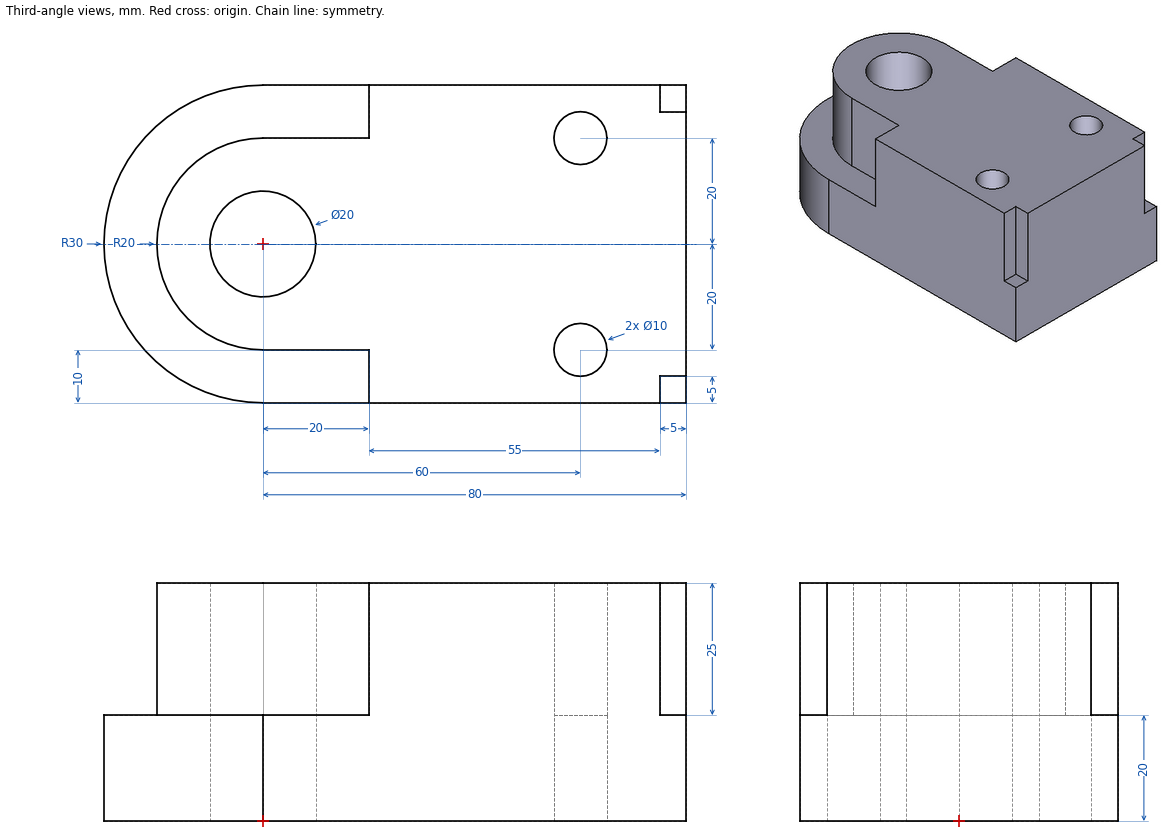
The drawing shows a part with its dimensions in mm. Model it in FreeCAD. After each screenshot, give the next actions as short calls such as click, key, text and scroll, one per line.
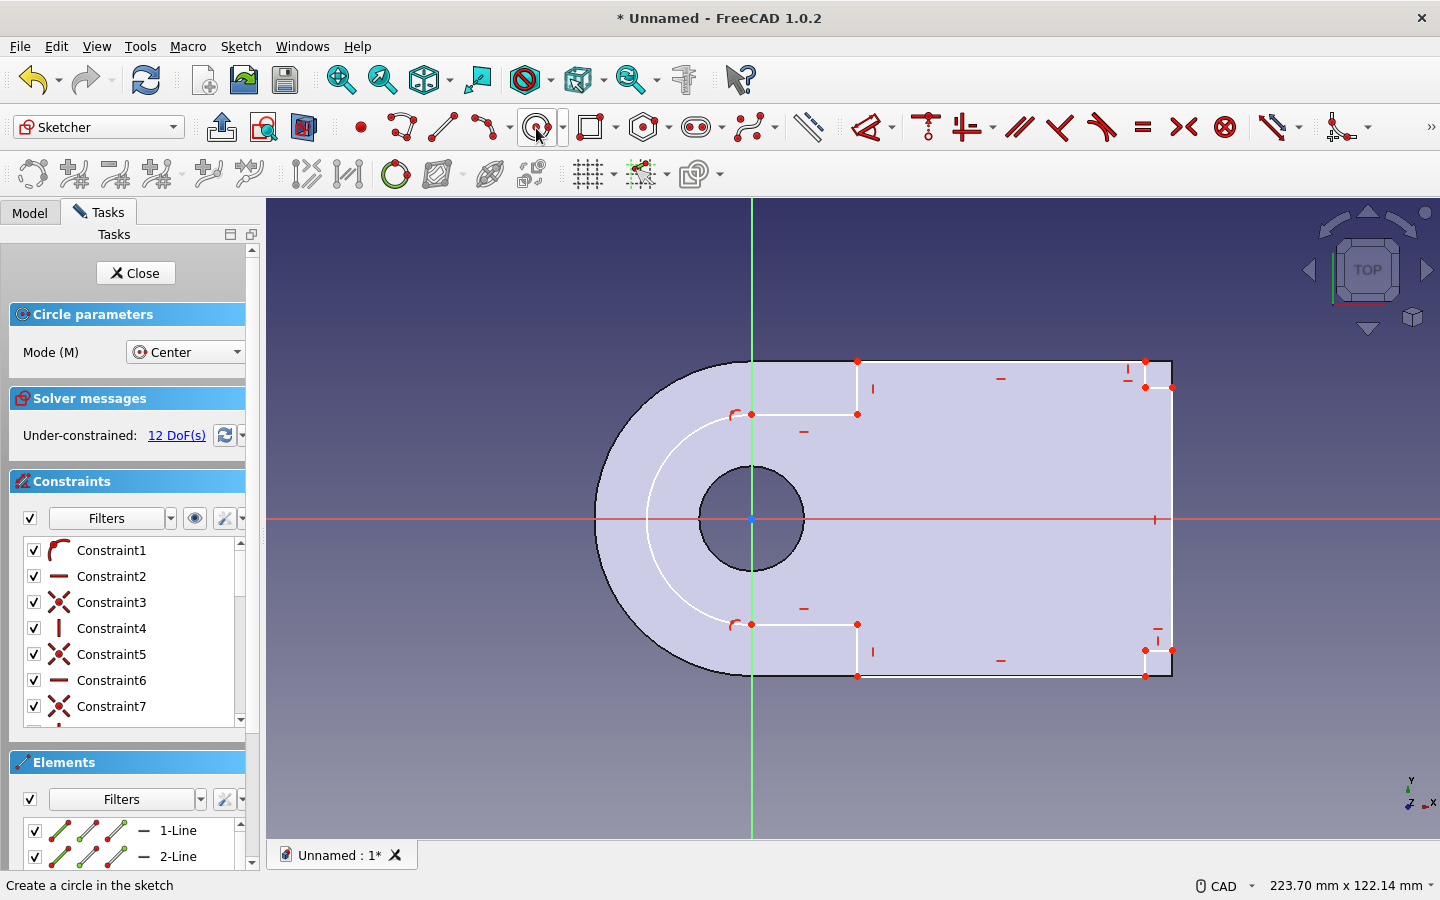
click(1067, 624)
move(1085, 605)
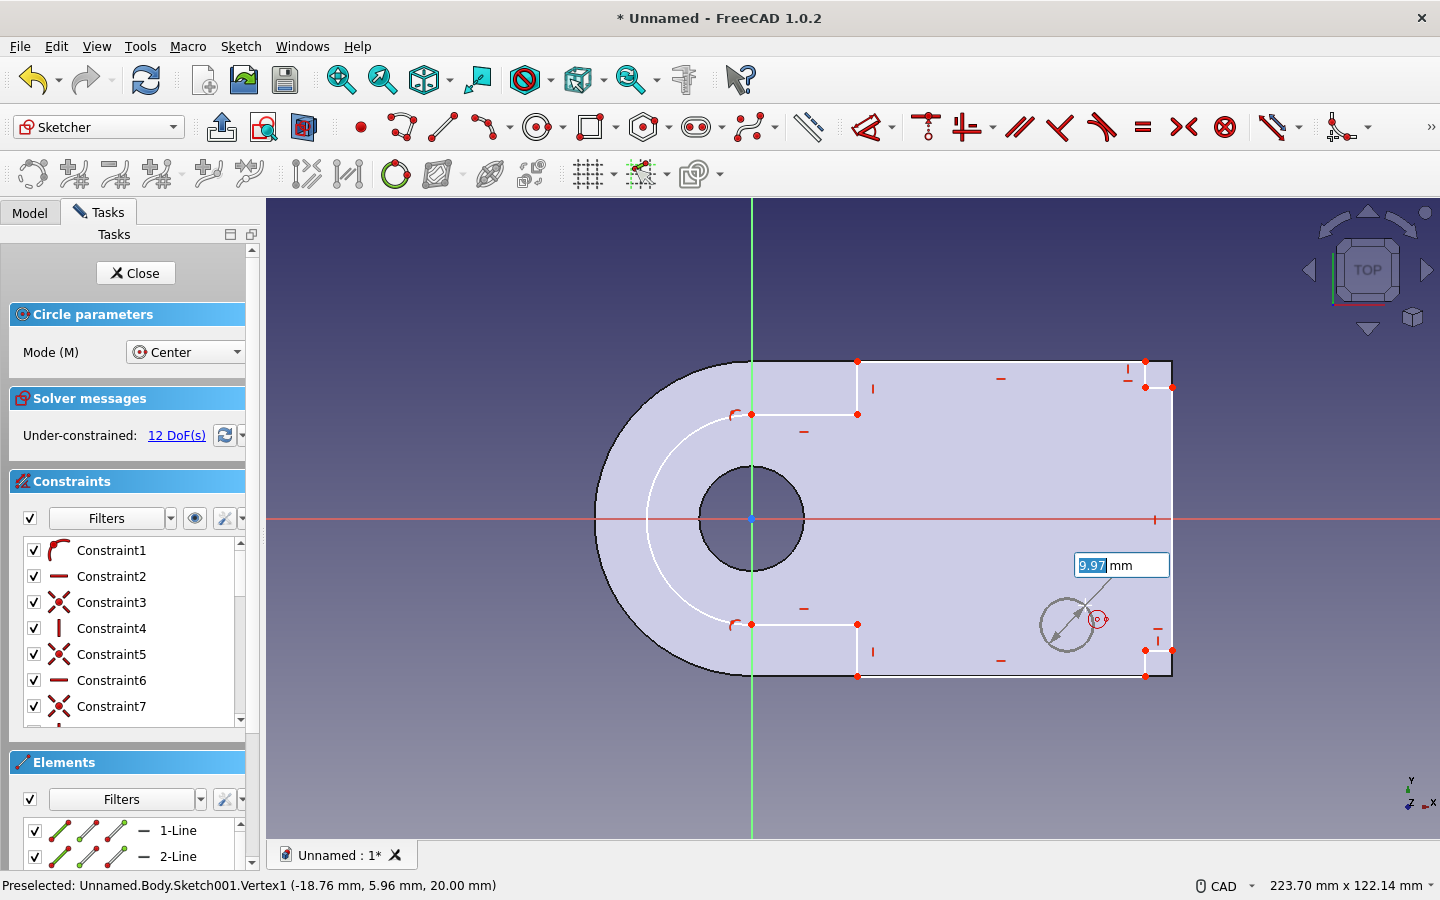
text(10)
key(Return)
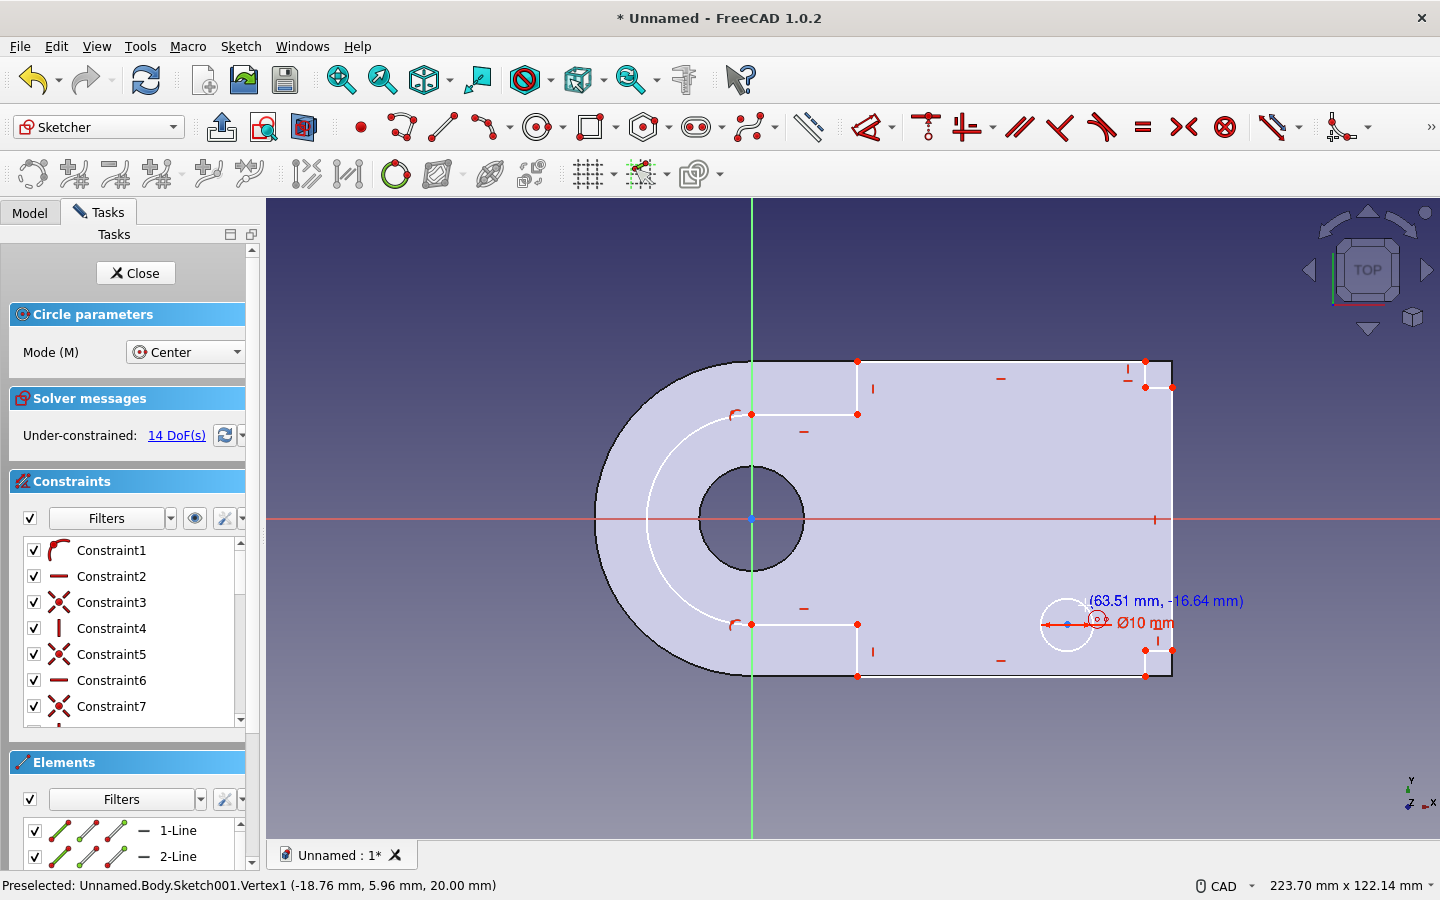
click(1067, 414)
move(1085, 395)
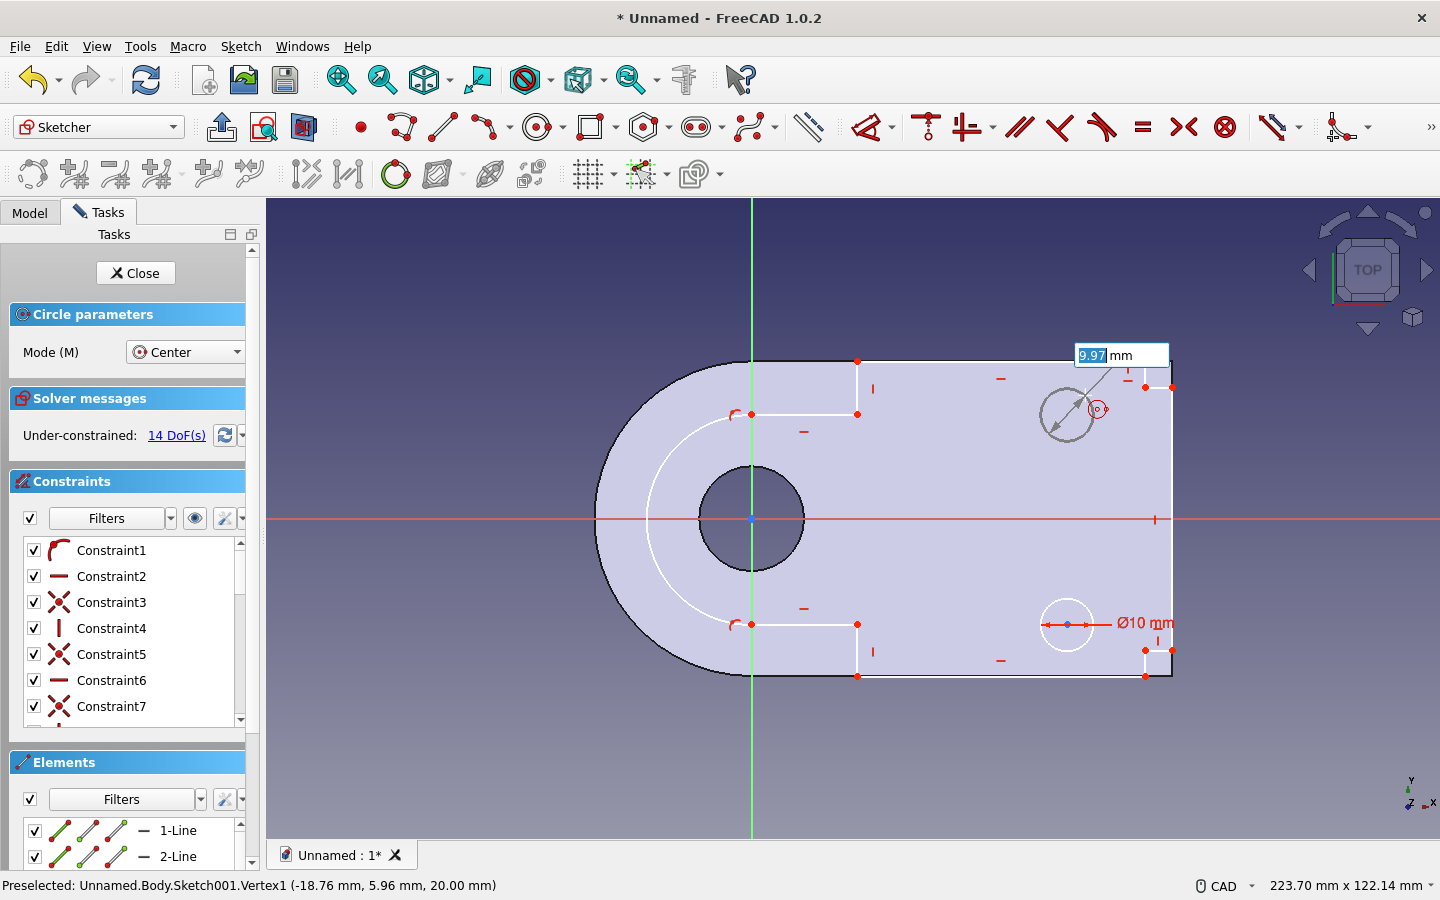
text(10)
key(Return)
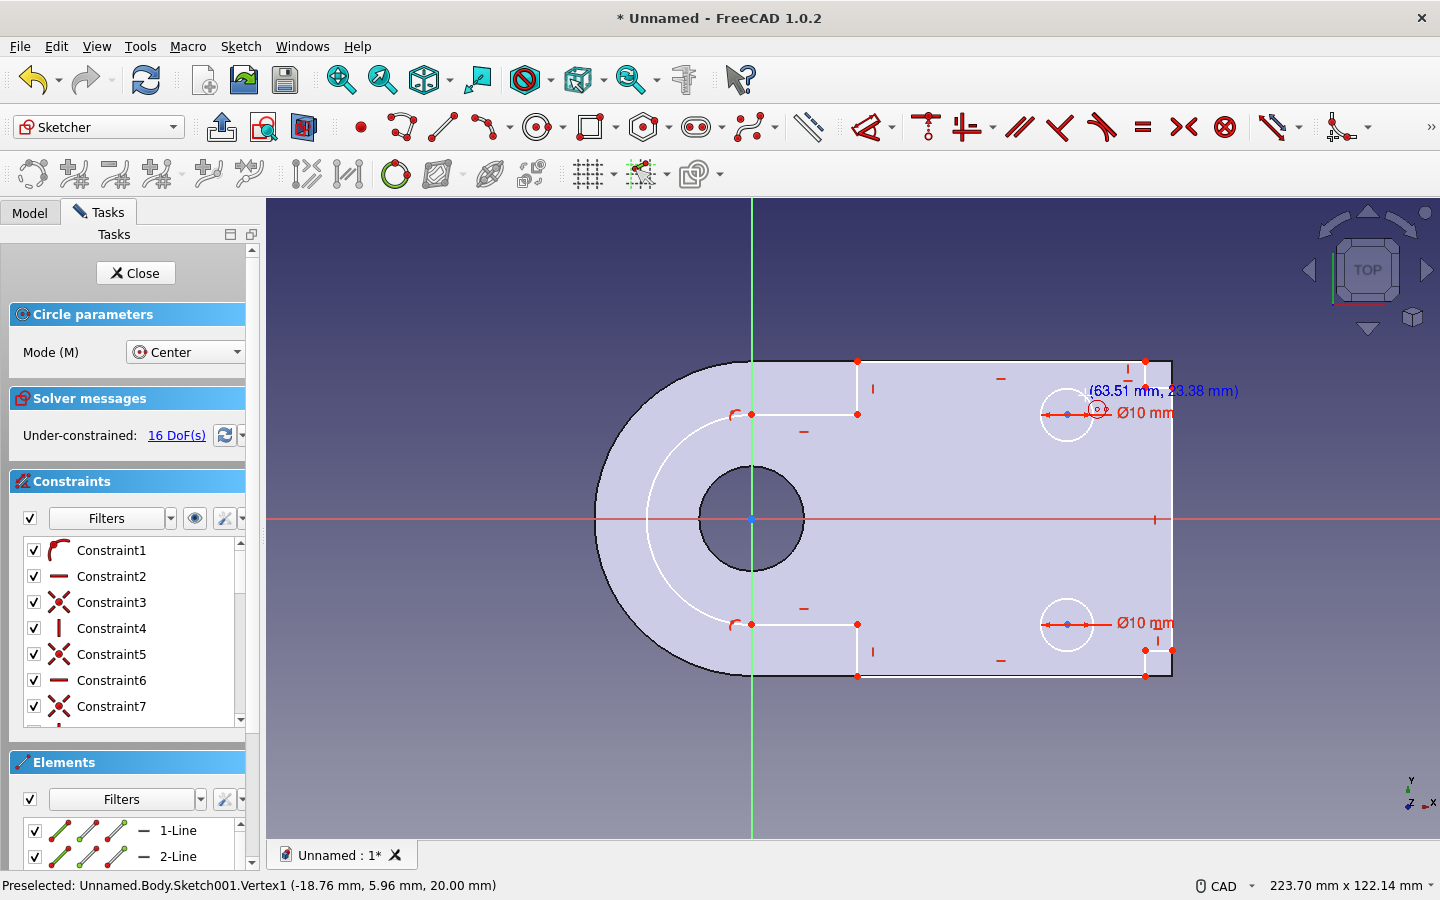
click(752, 519)
move(789, 482)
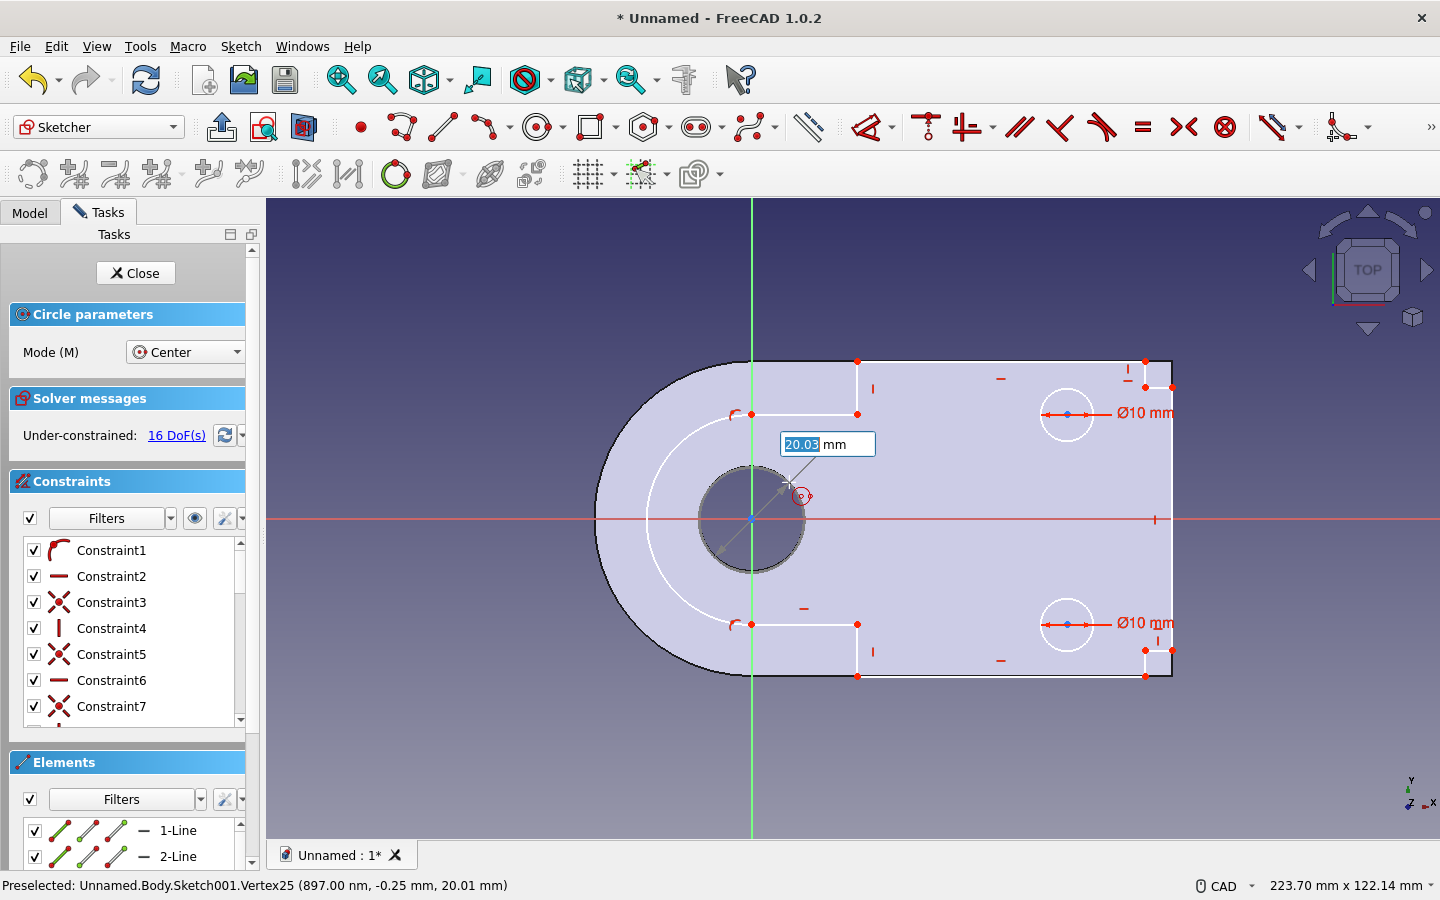
text(20)
key(Return)
key(Escape)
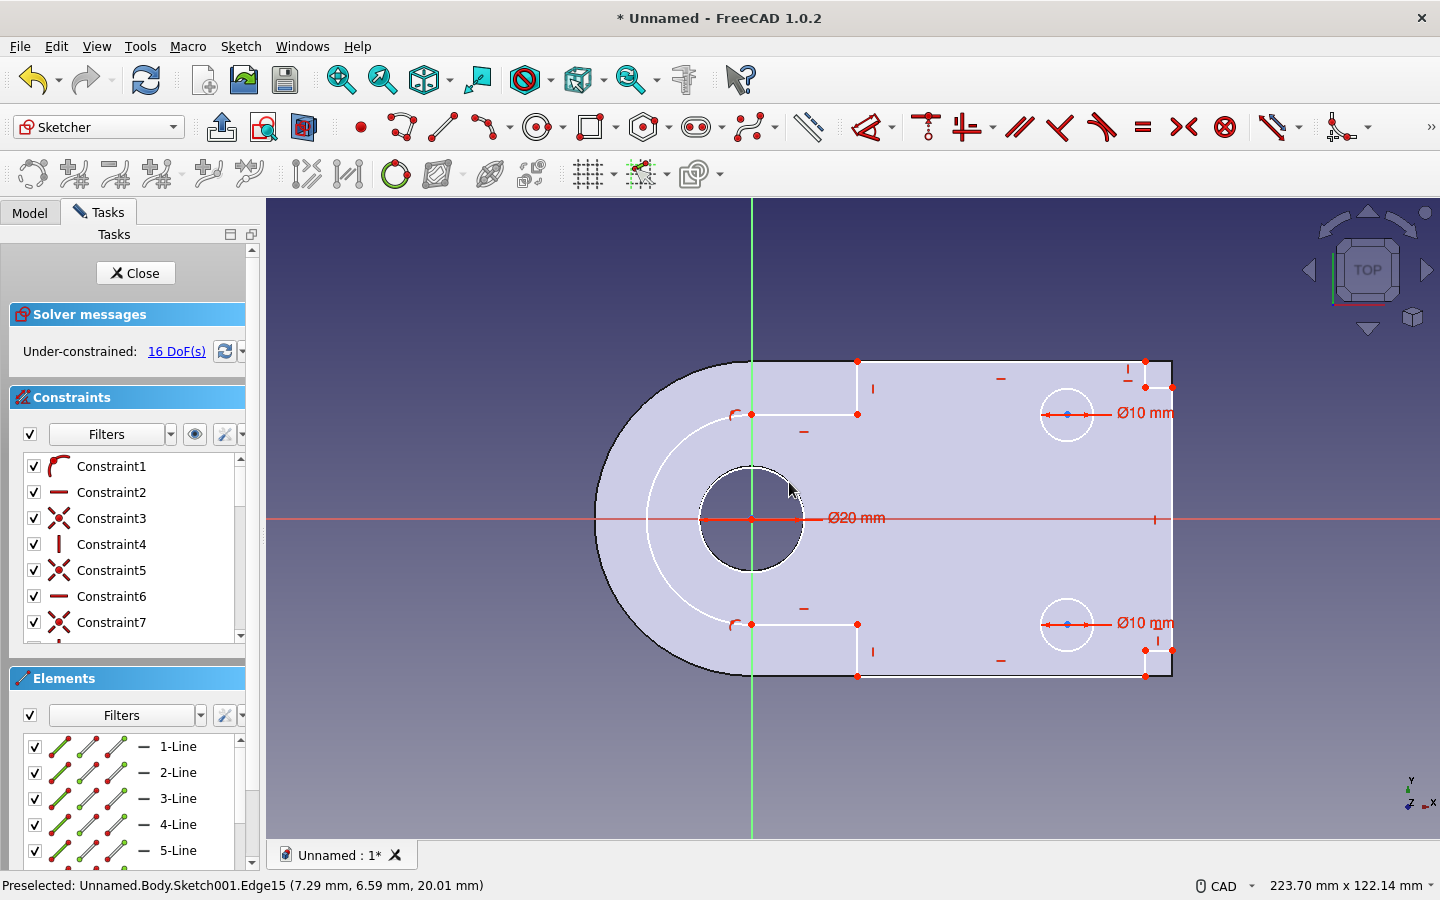
click(783, 625)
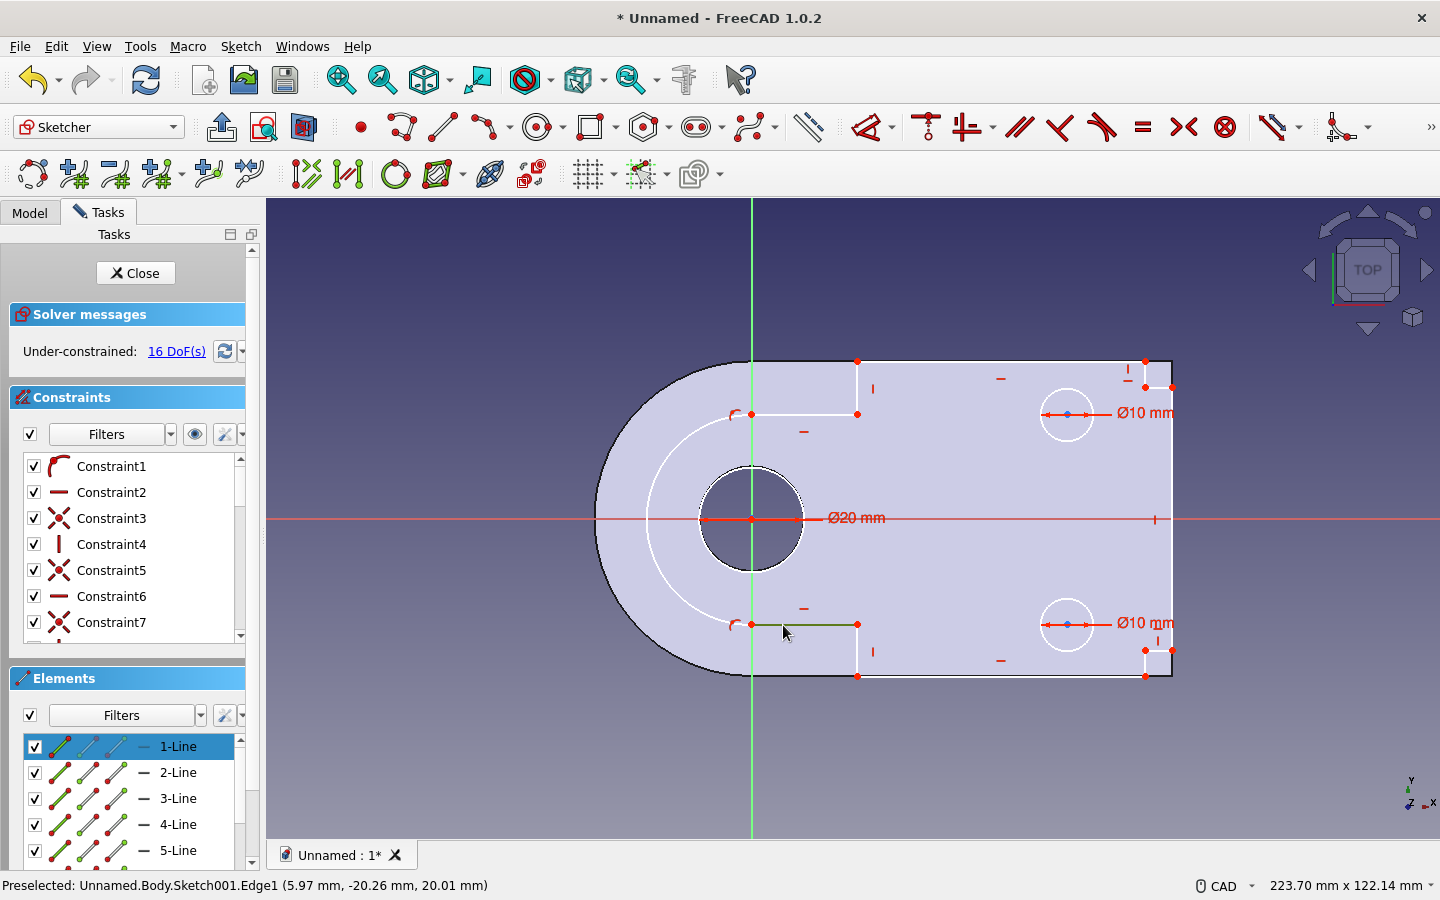
click(667, 458)